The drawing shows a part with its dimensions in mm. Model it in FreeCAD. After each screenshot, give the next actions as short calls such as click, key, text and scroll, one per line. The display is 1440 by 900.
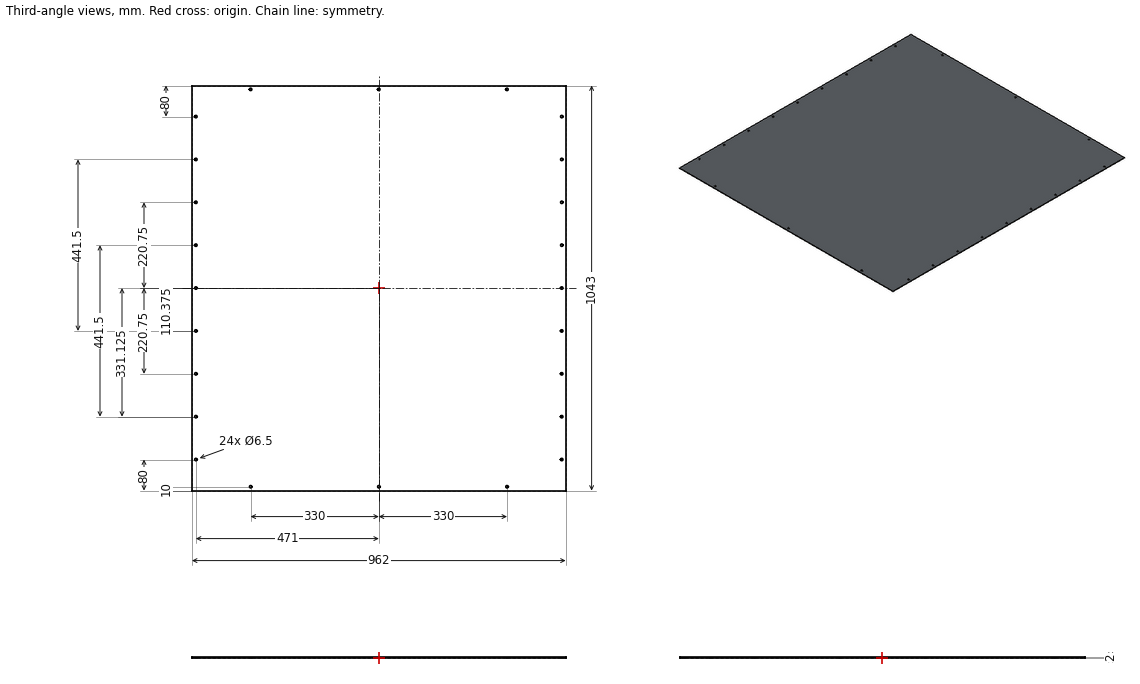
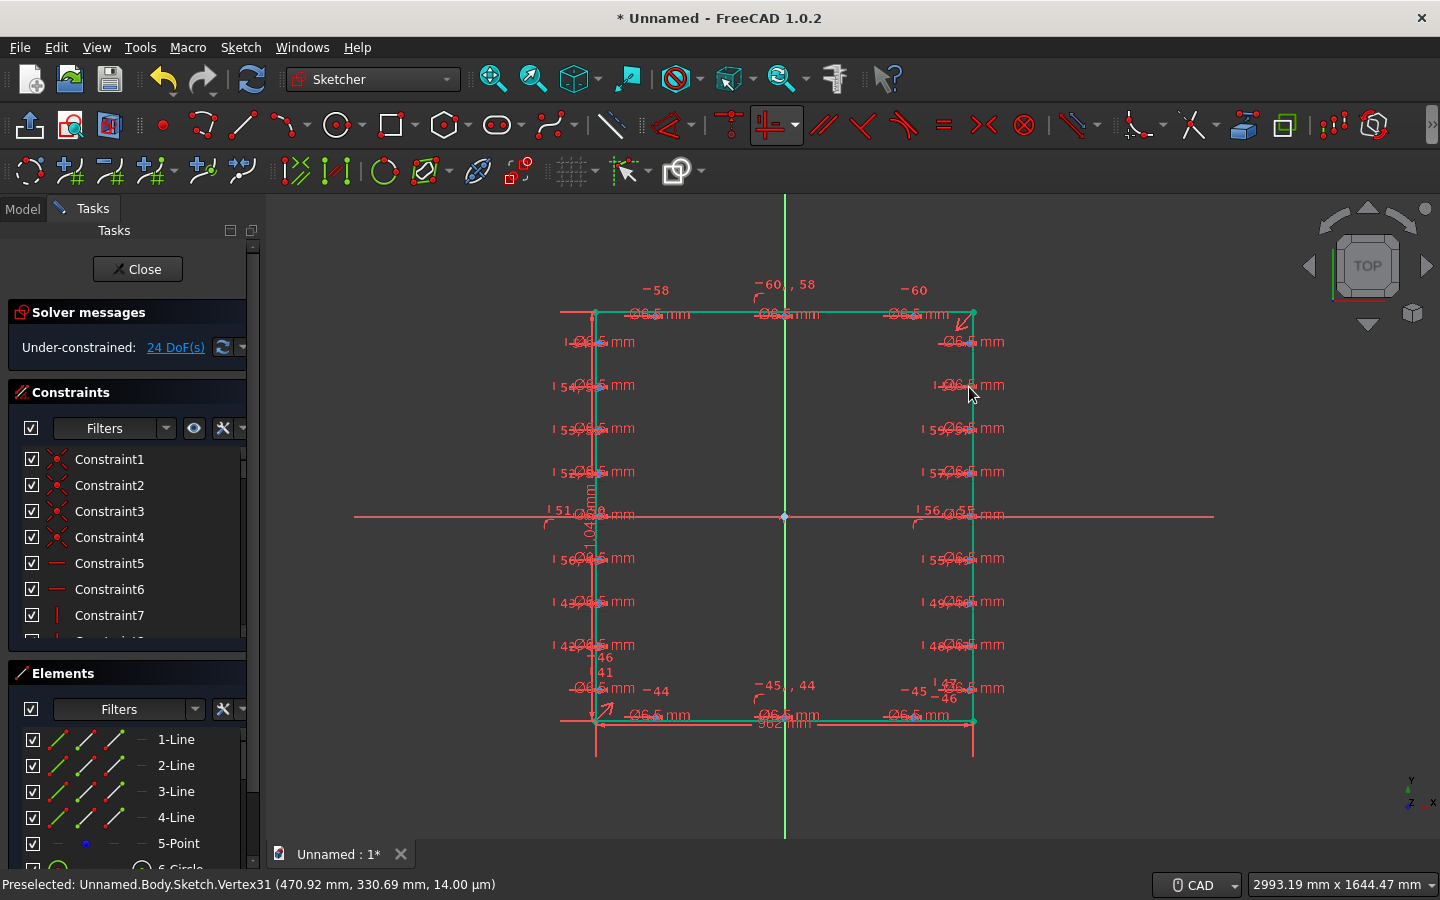
click(969, 344)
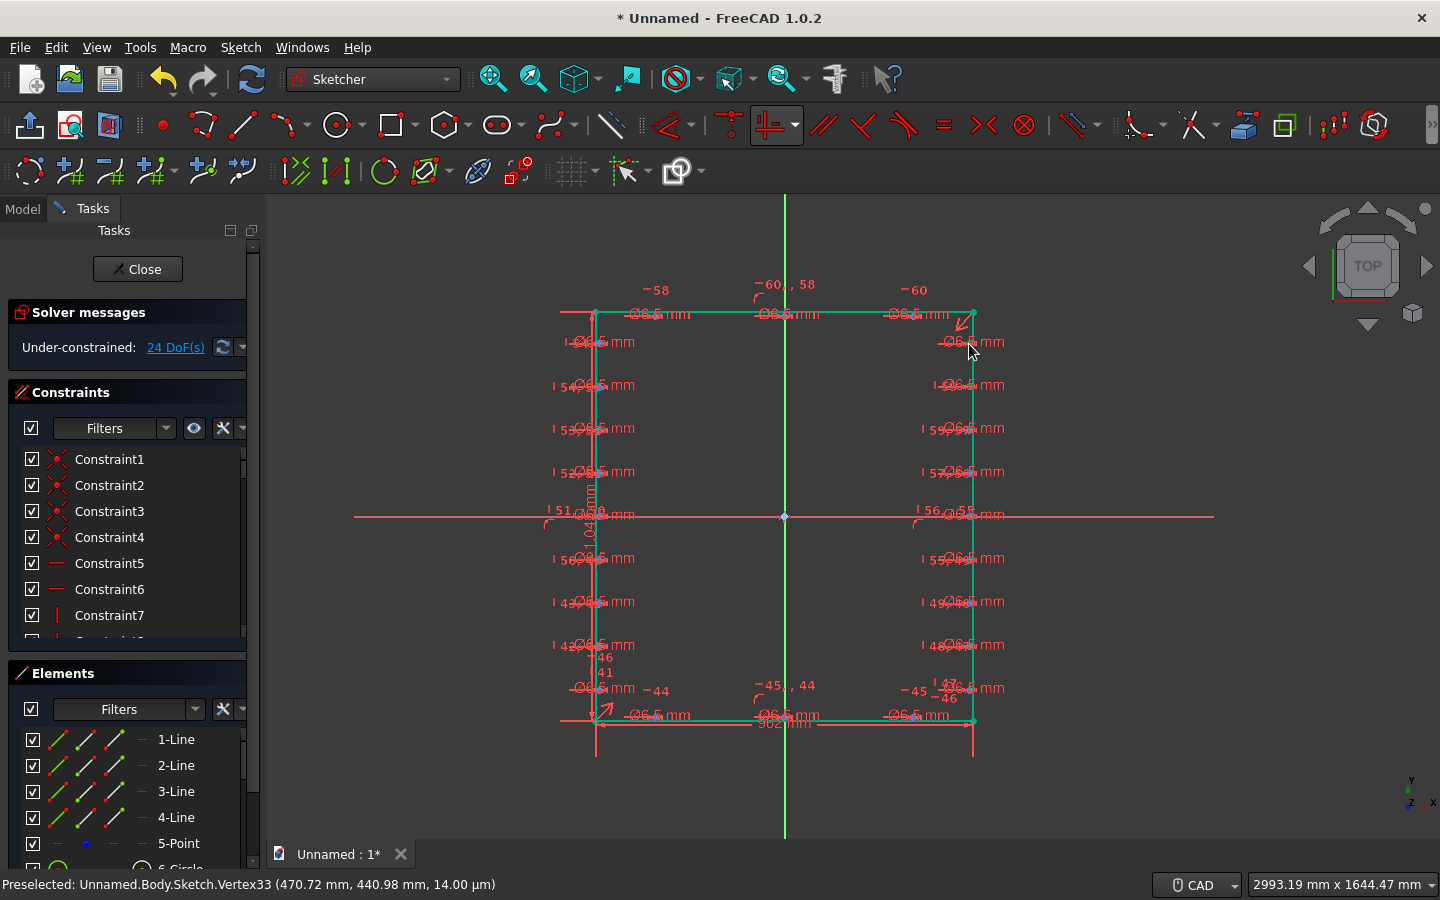
click(798, 126)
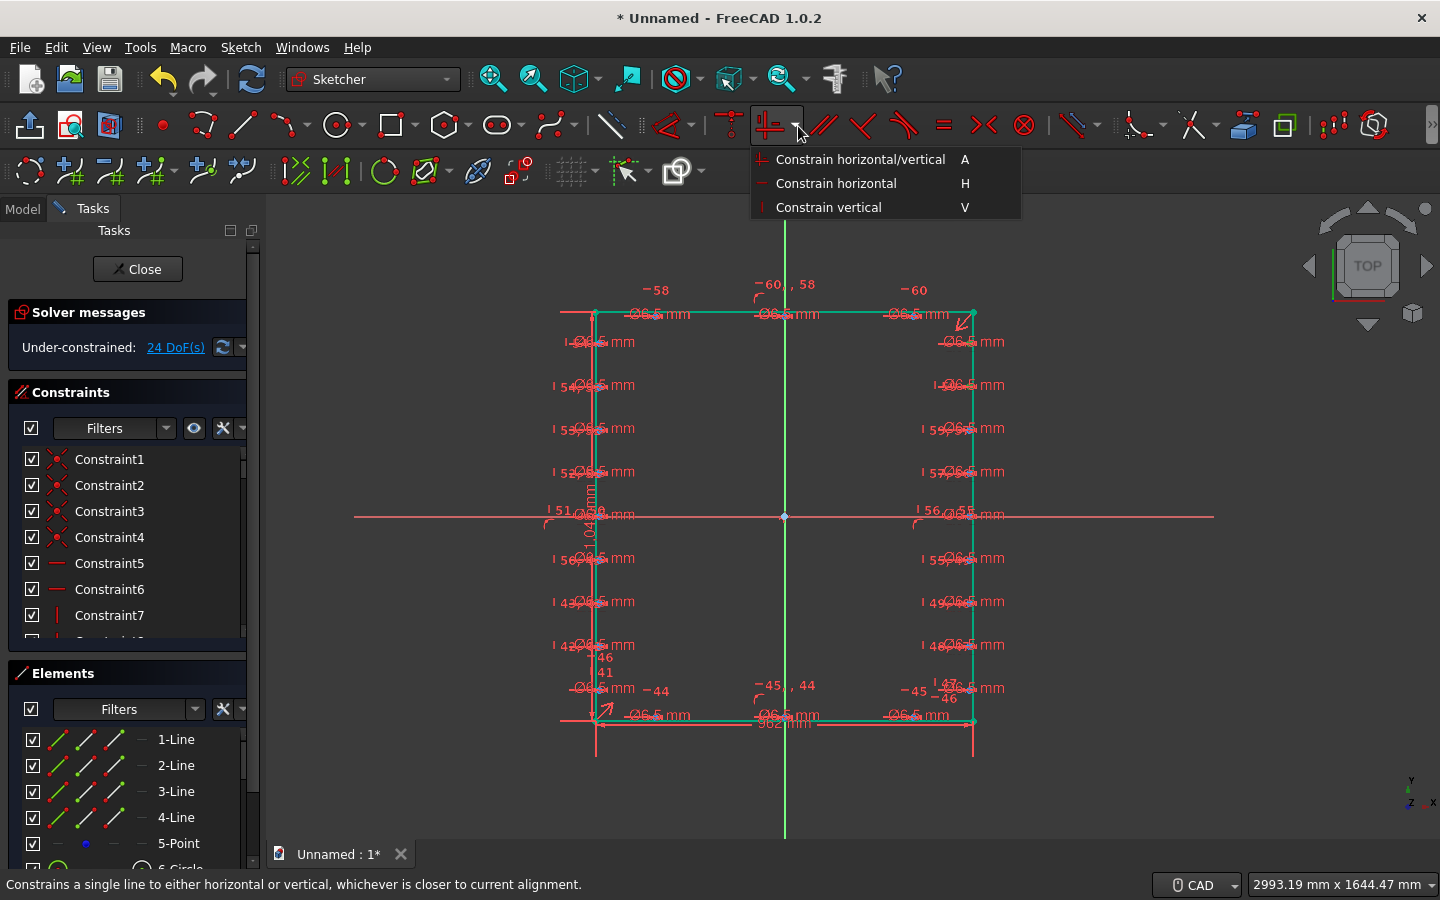
click(886, 207)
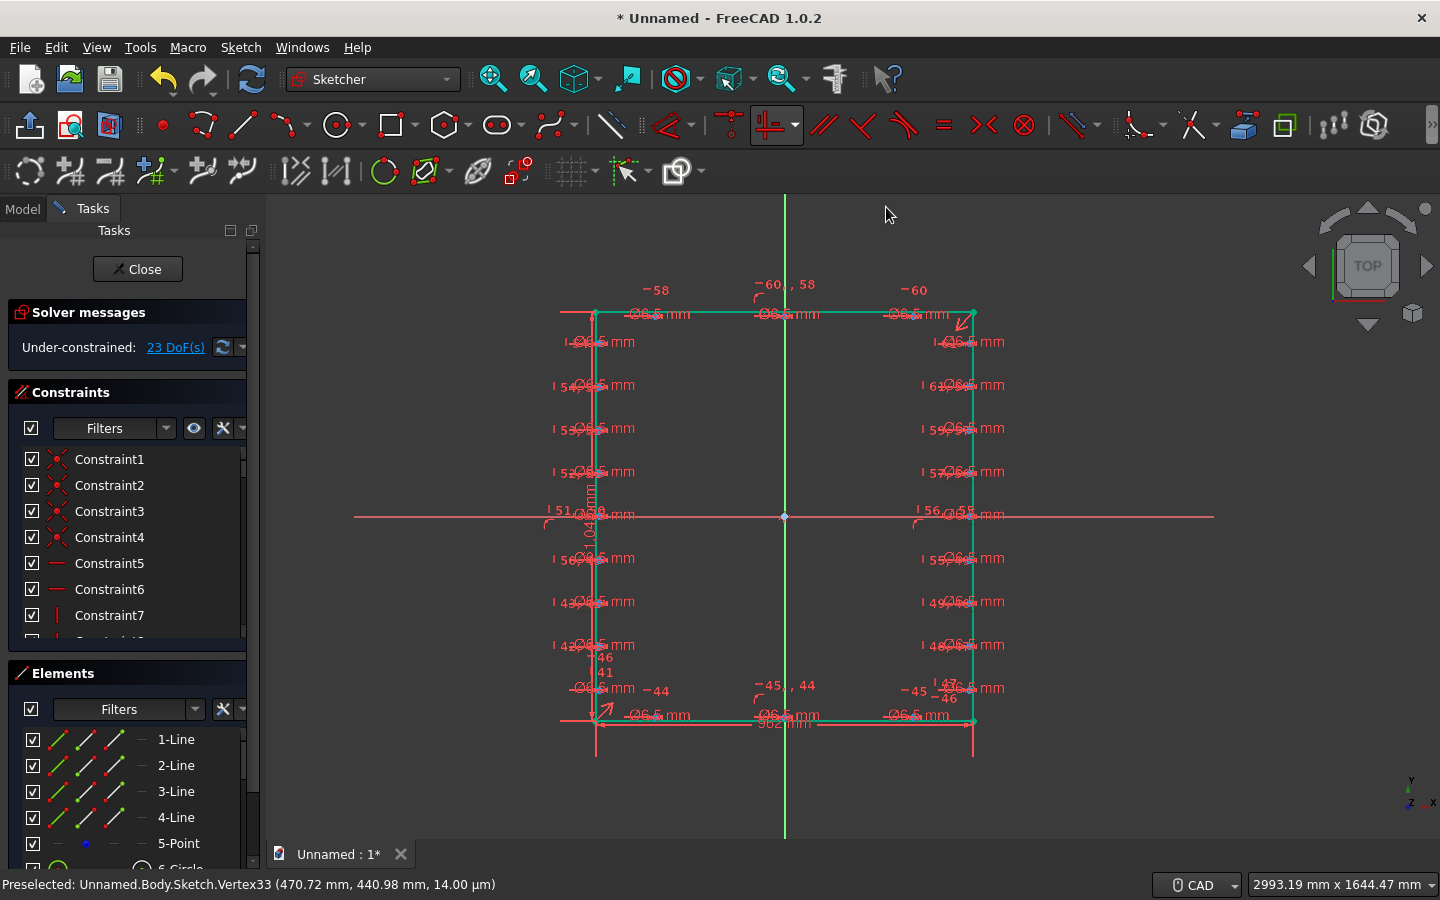
click(600, 647)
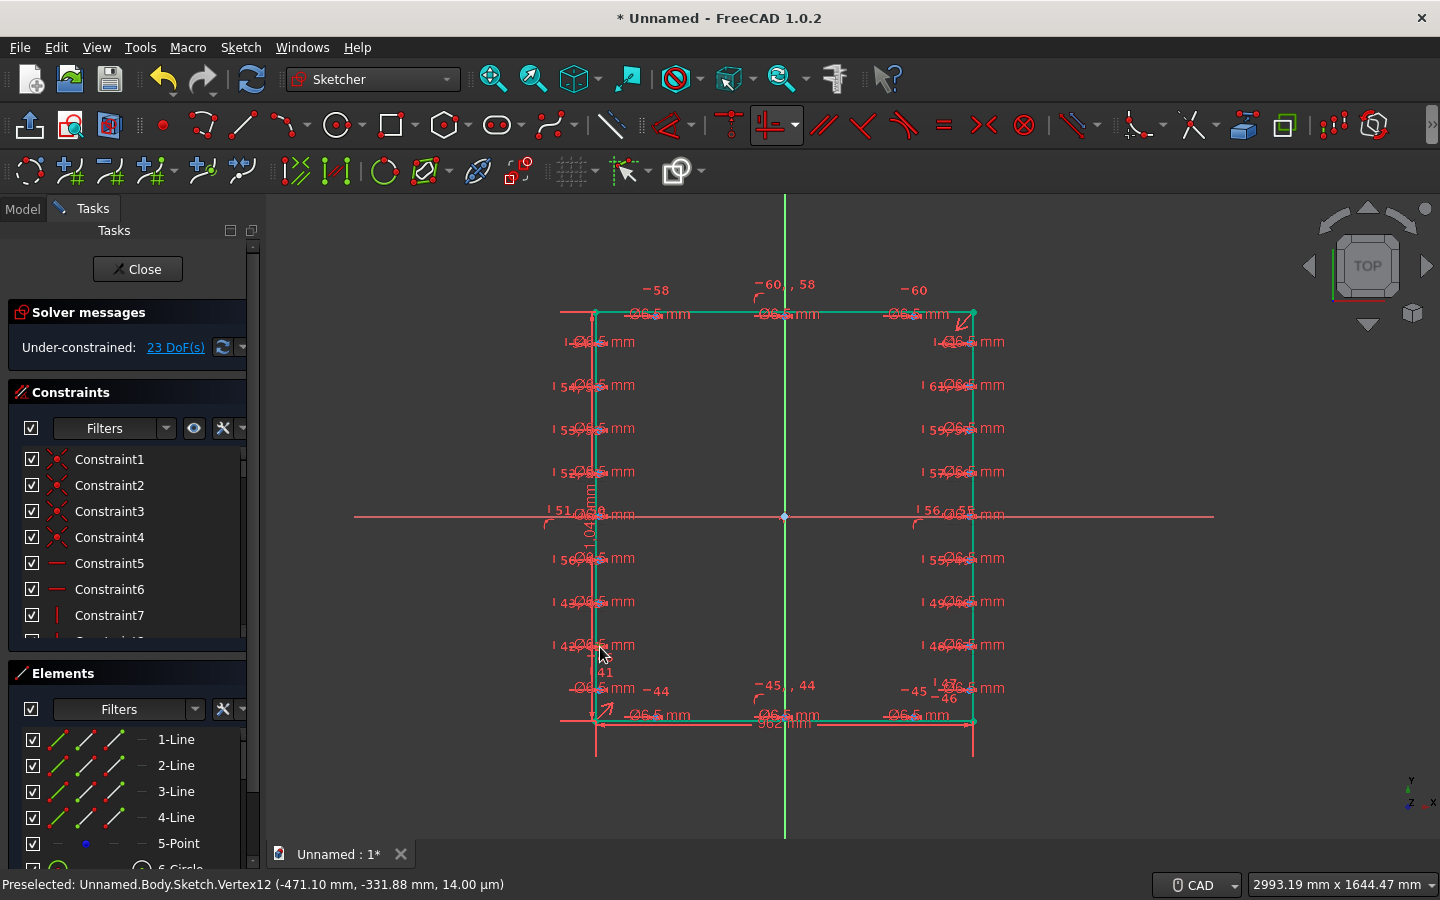
click(969, 647)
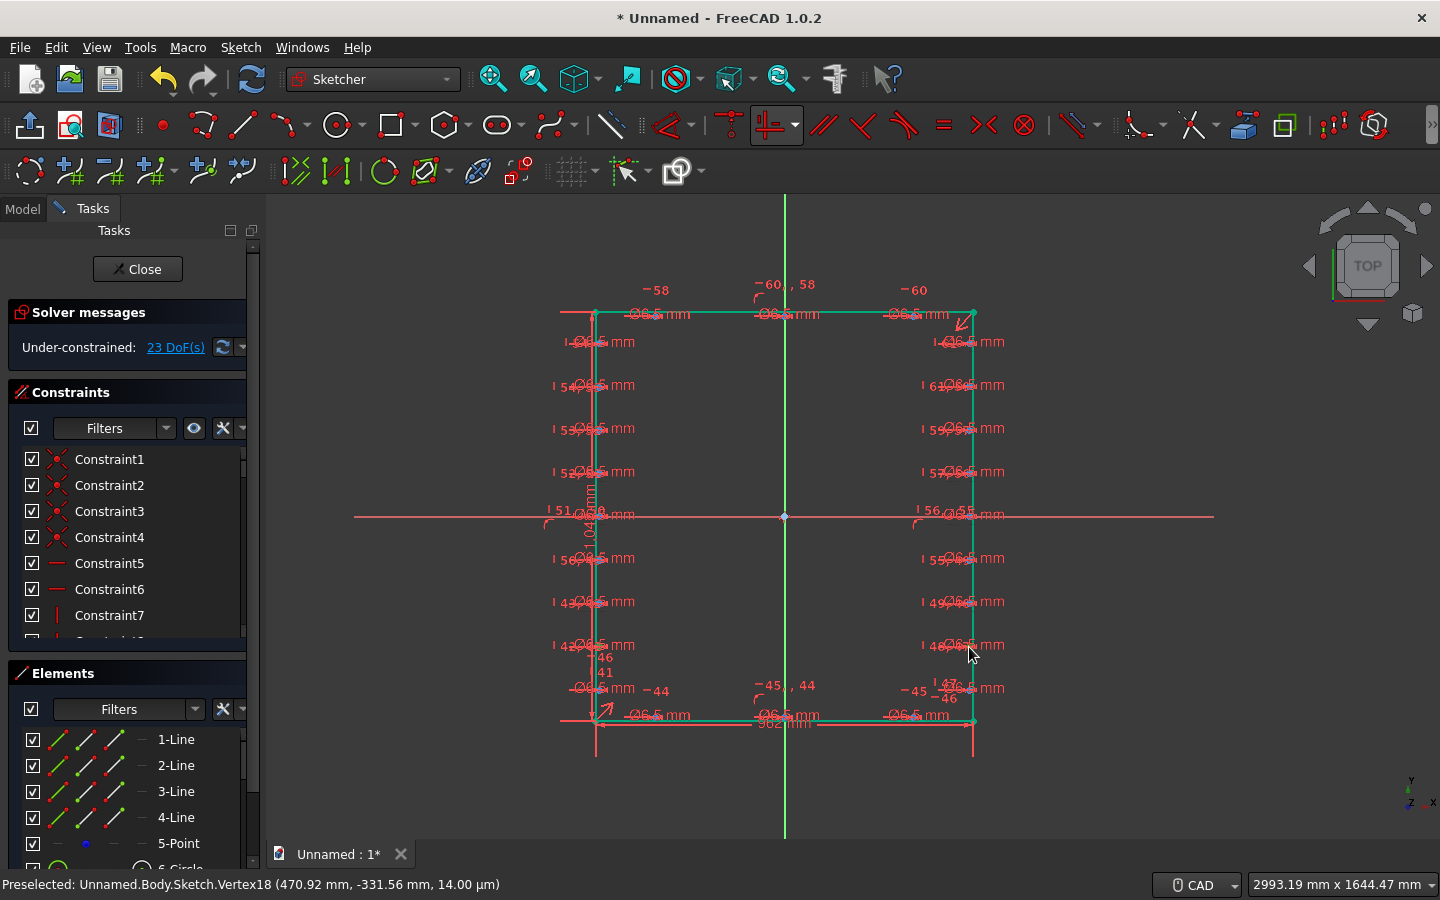
click(785, 769)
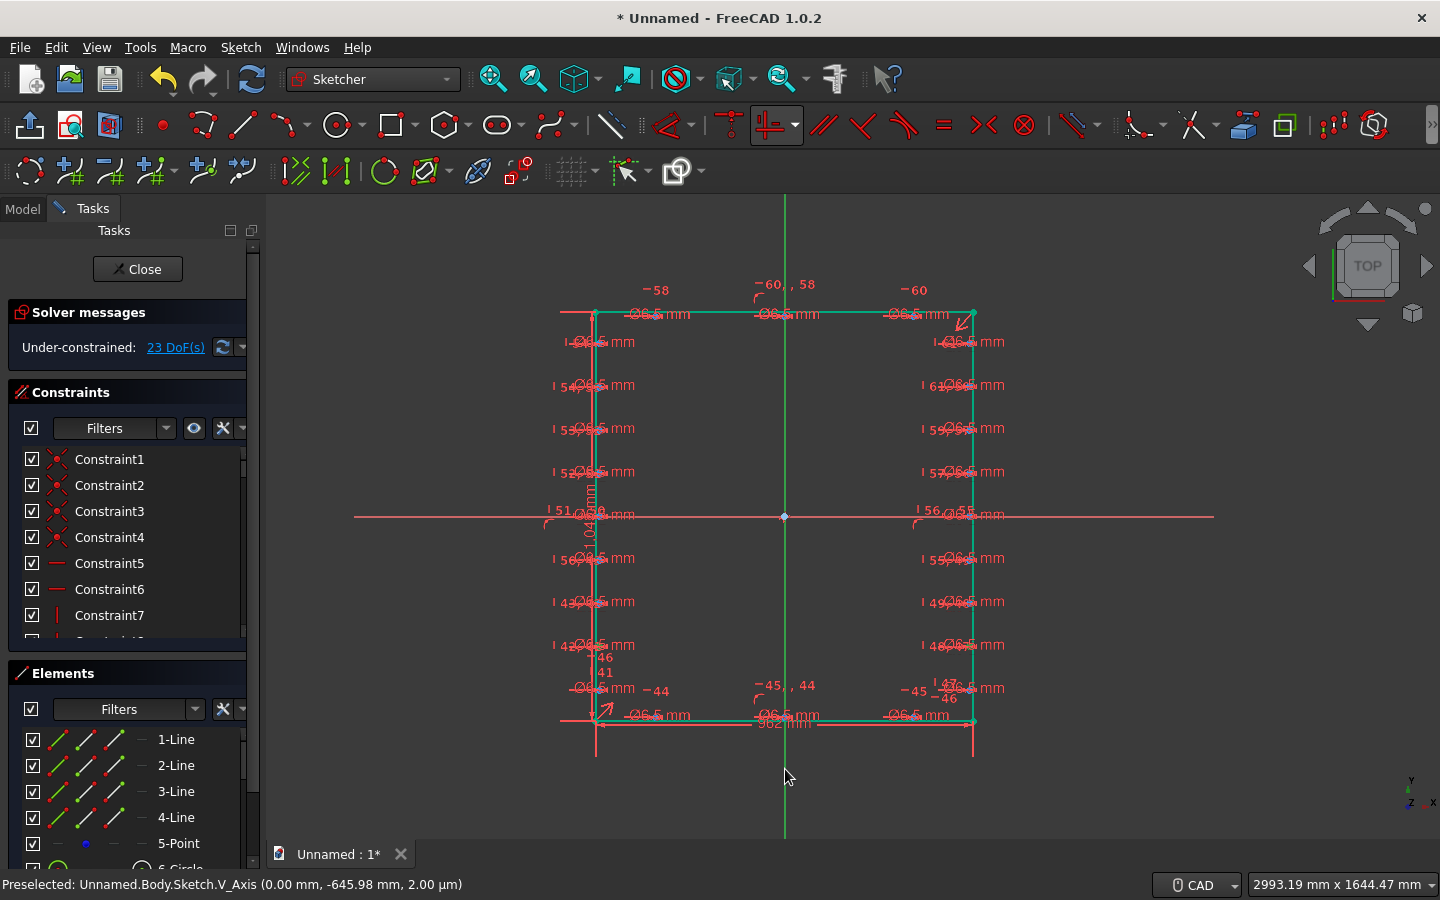
click(984, 126)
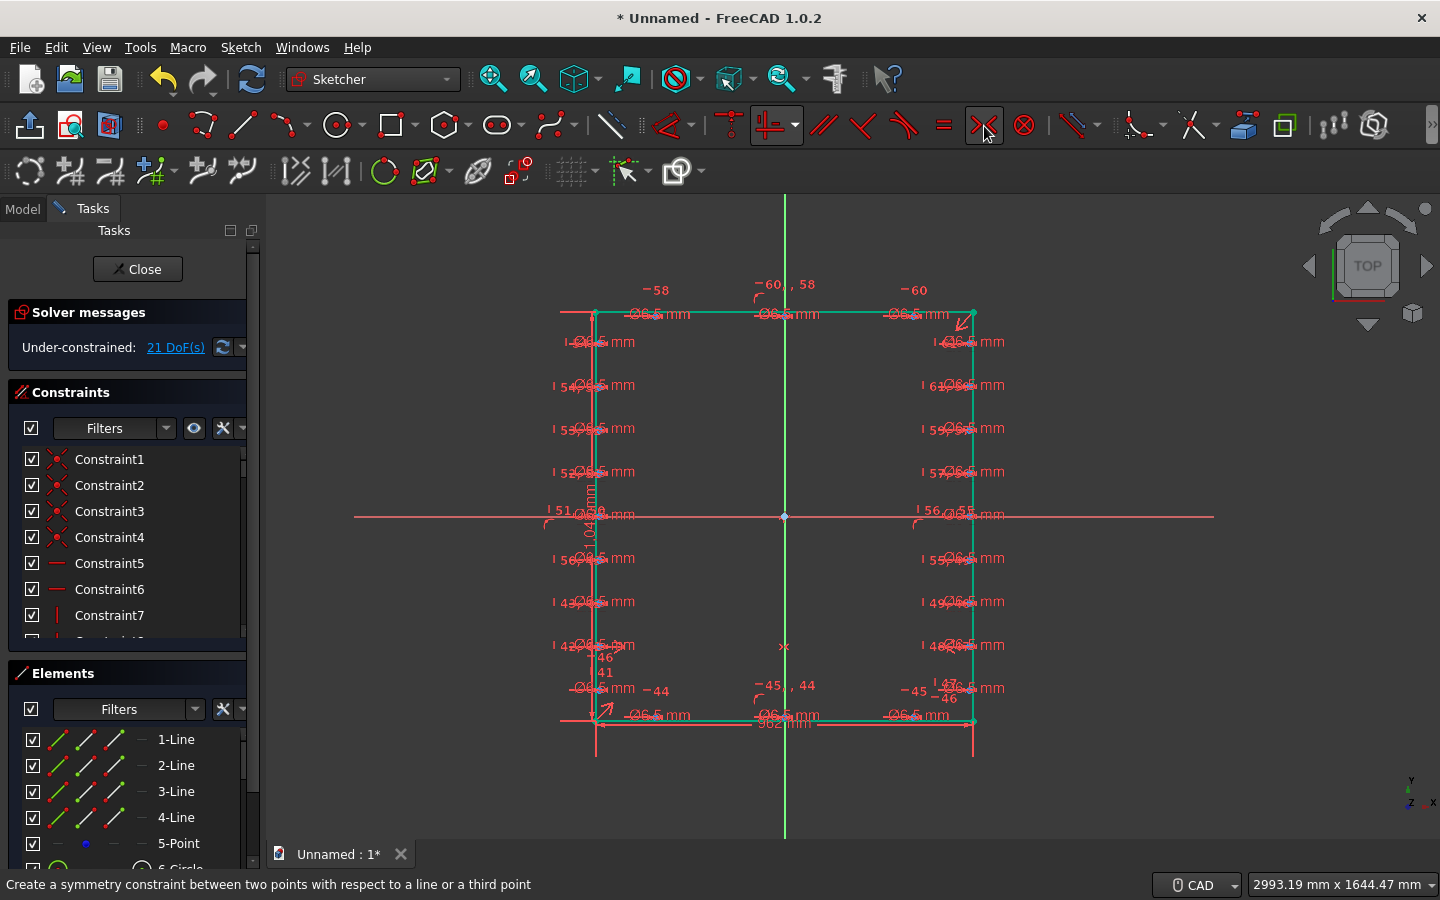
click(655, 717)